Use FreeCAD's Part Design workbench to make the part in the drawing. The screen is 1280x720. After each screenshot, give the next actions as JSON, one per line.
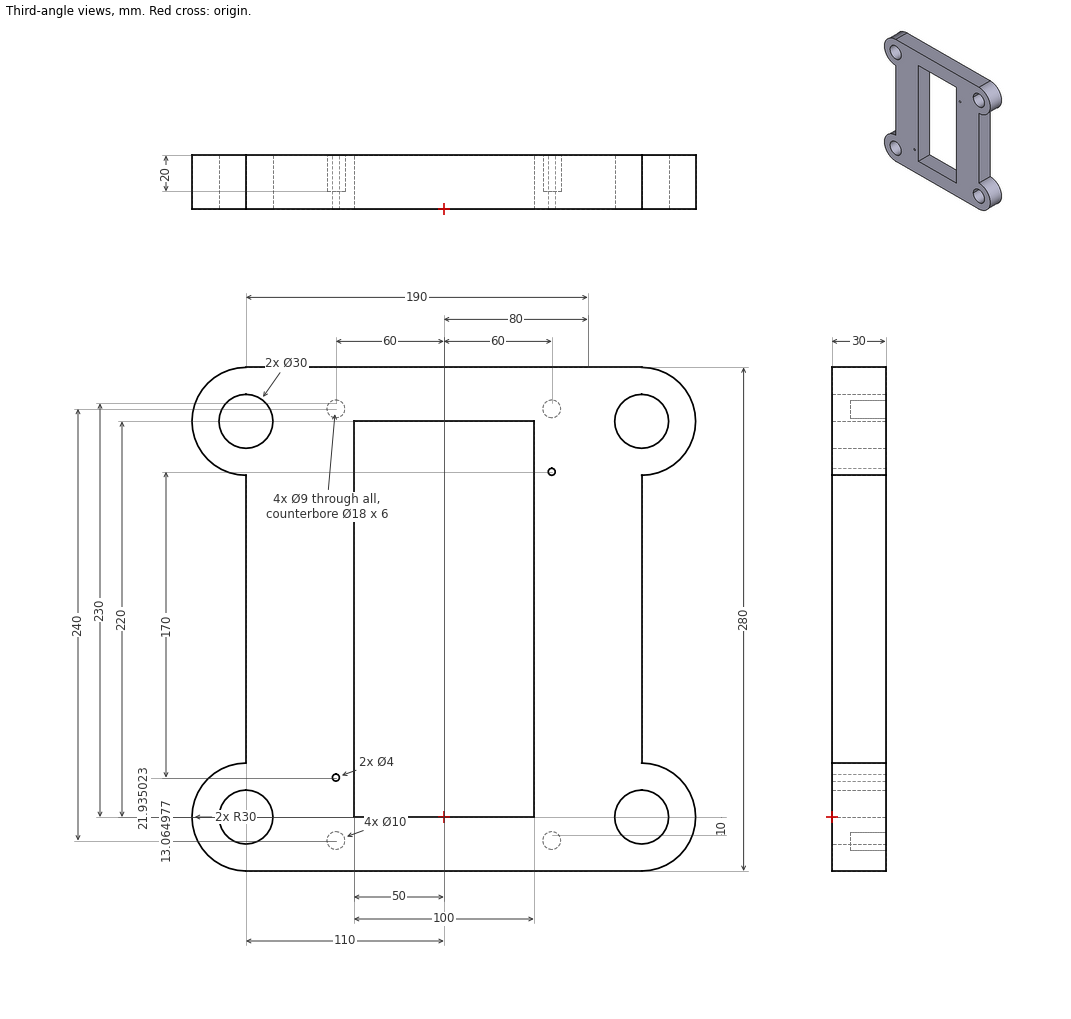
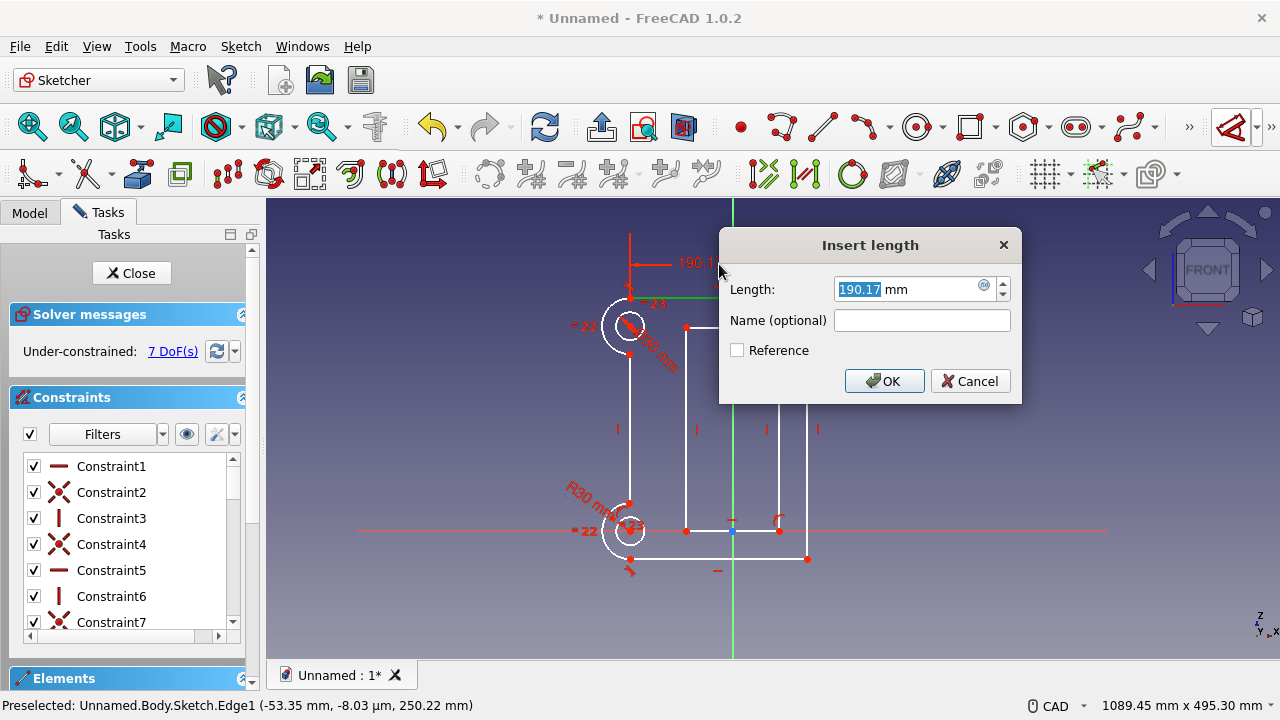
{"action": "type", "text": "190"}
{"action": "key", "text": "Return"}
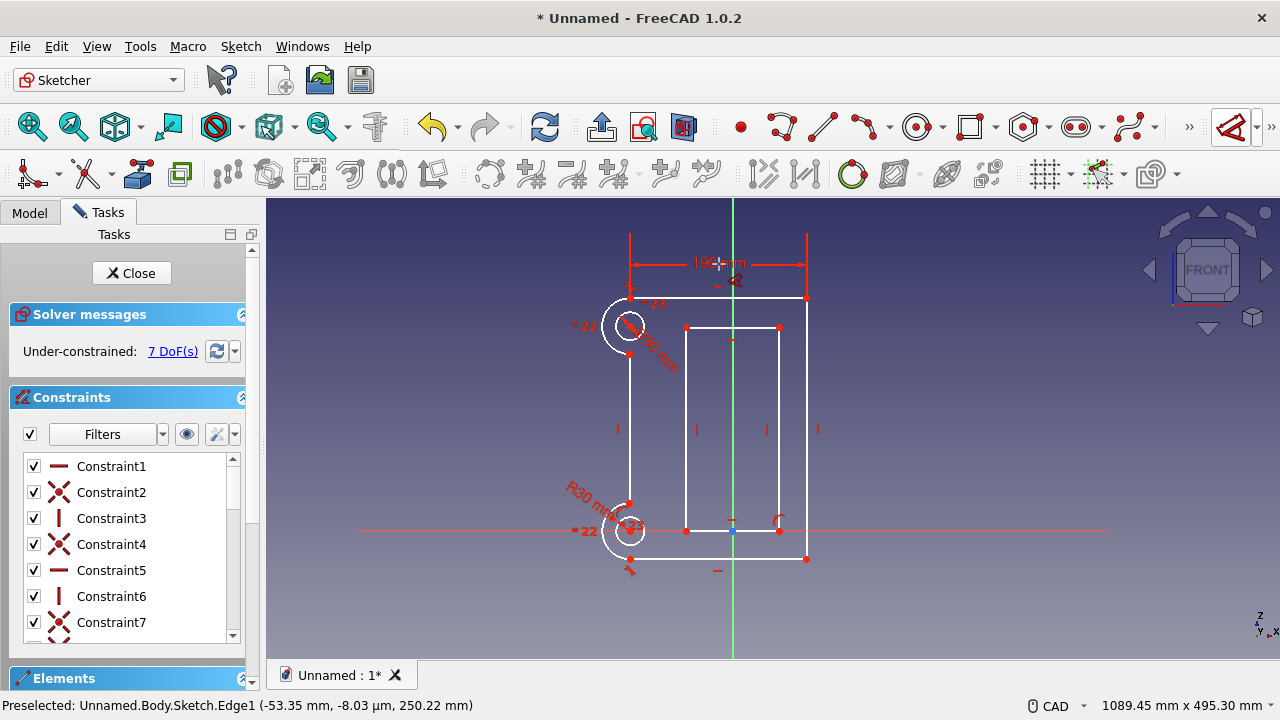
{"action": "left_click", "coordinate": [807, 377]}
{"action": "left_click", "coordinate": [841, 429]}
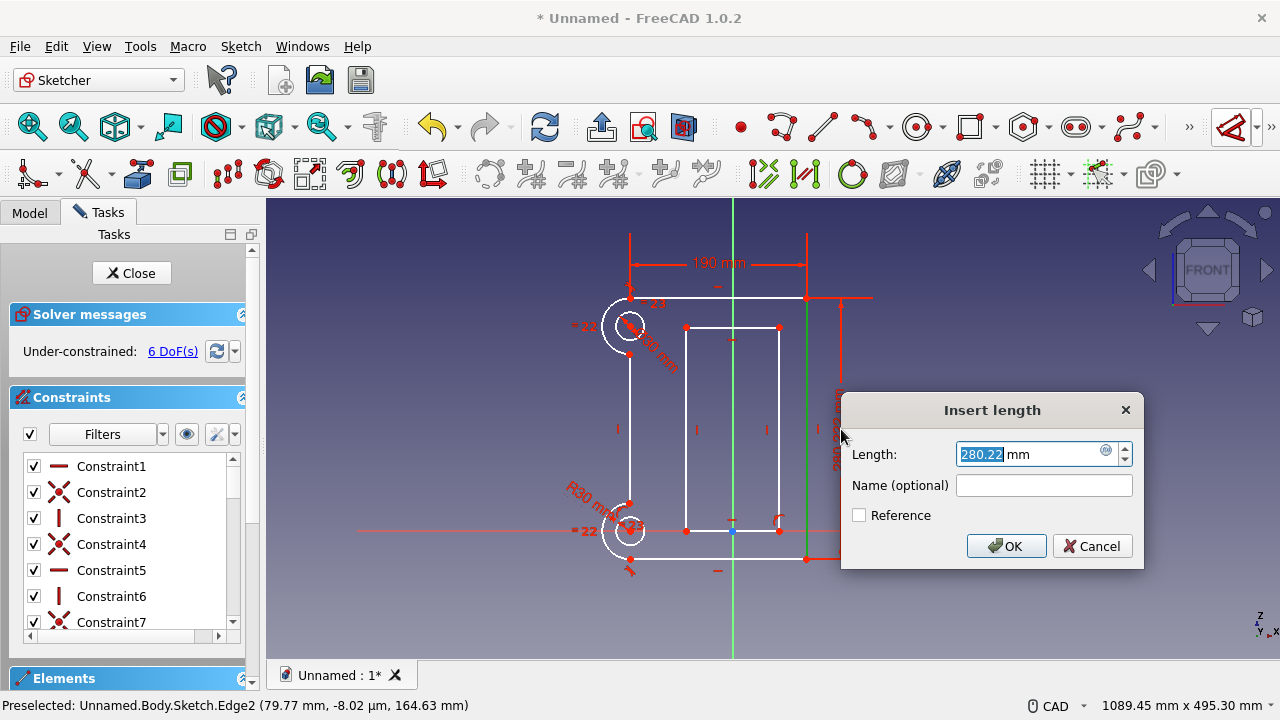
{"action": "type", "text": "280"}
{"action": "key", "text": "Return"}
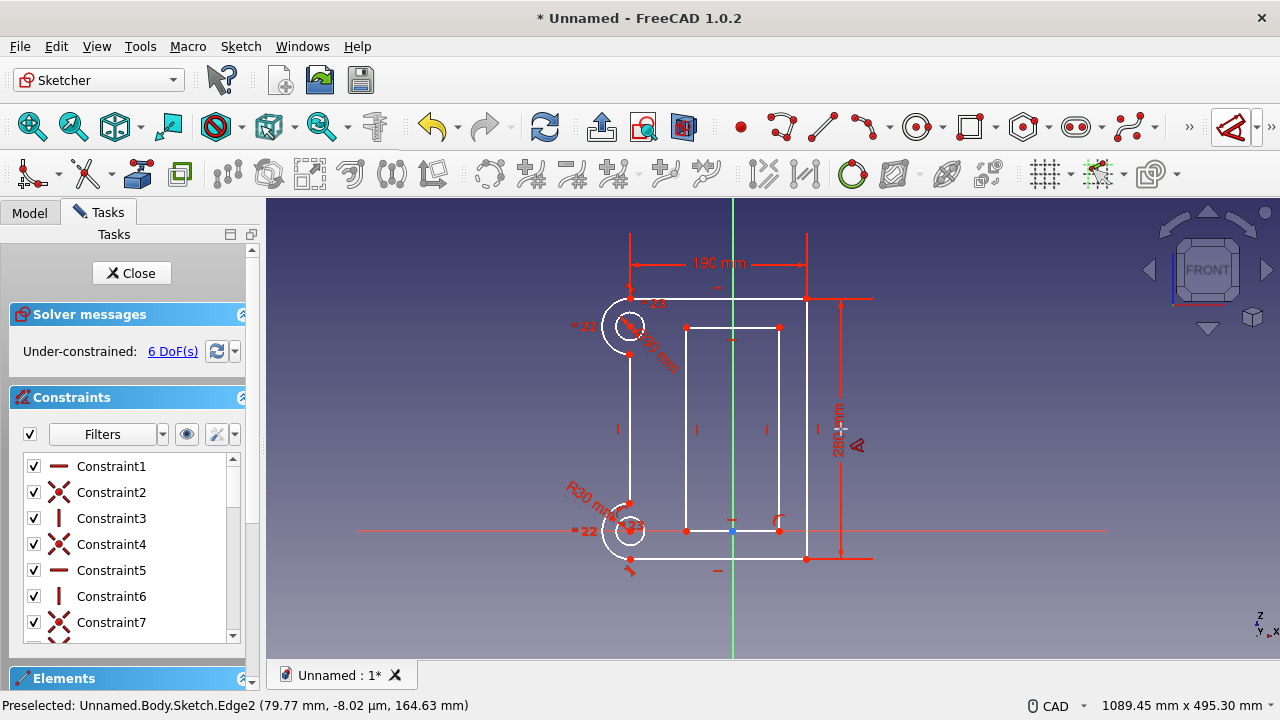
{"action": "left_click", "coordinate": [754, 559]}
{"action": "left_click", "coordinate": [719, 593]}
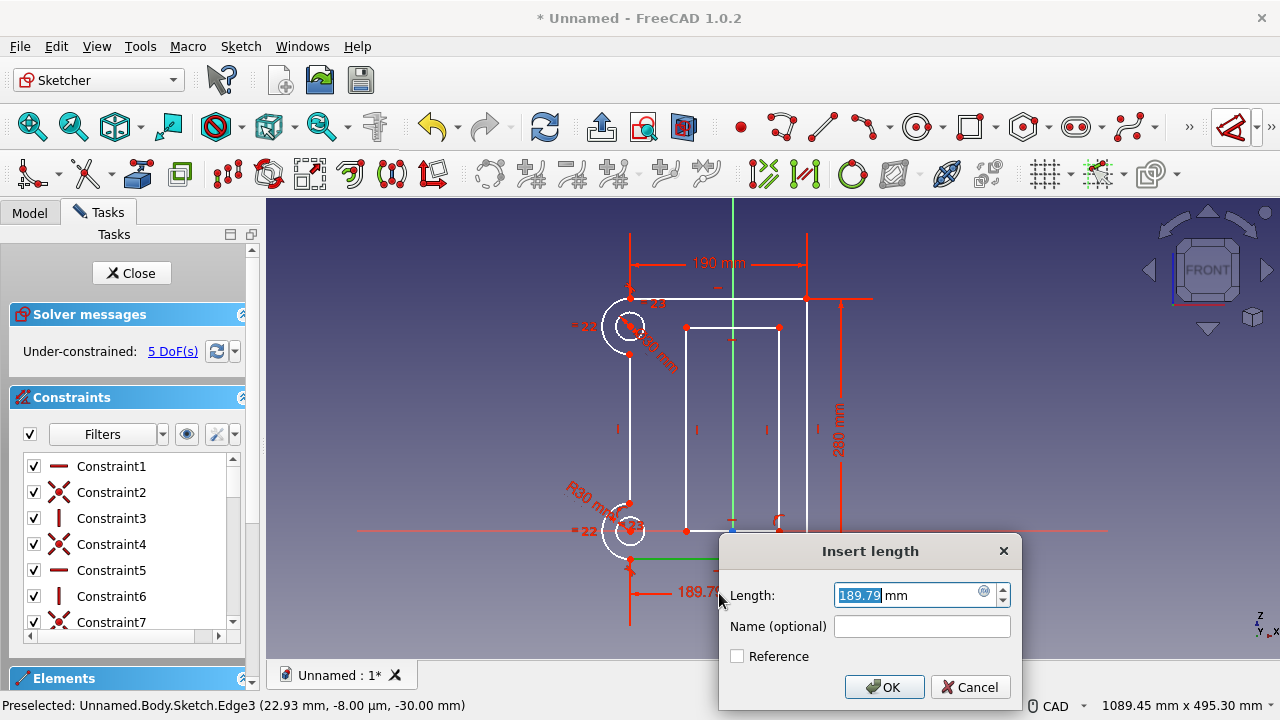
{"action": "type", "text": "190"}
{"action": "key", "text": "Return"}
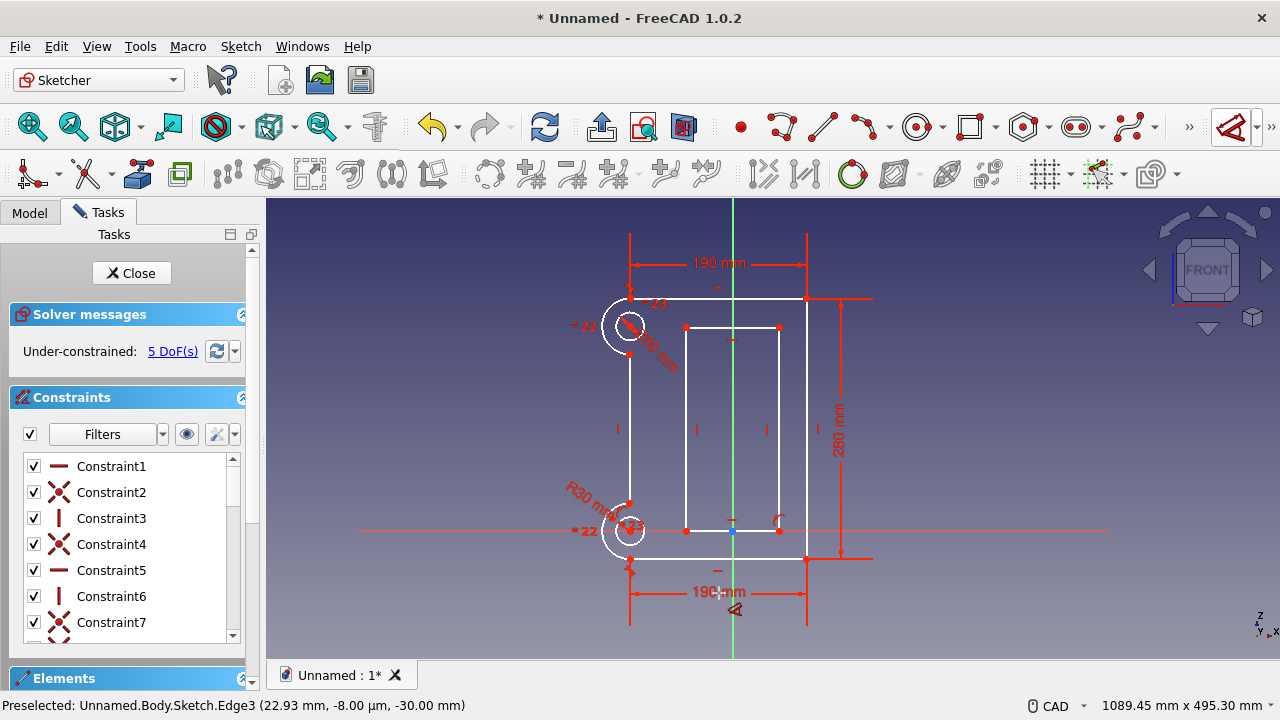
{"action": "left_click", "coordinate": [686, 389]}
{"action": "left_click", "coordinate": [652, 429]}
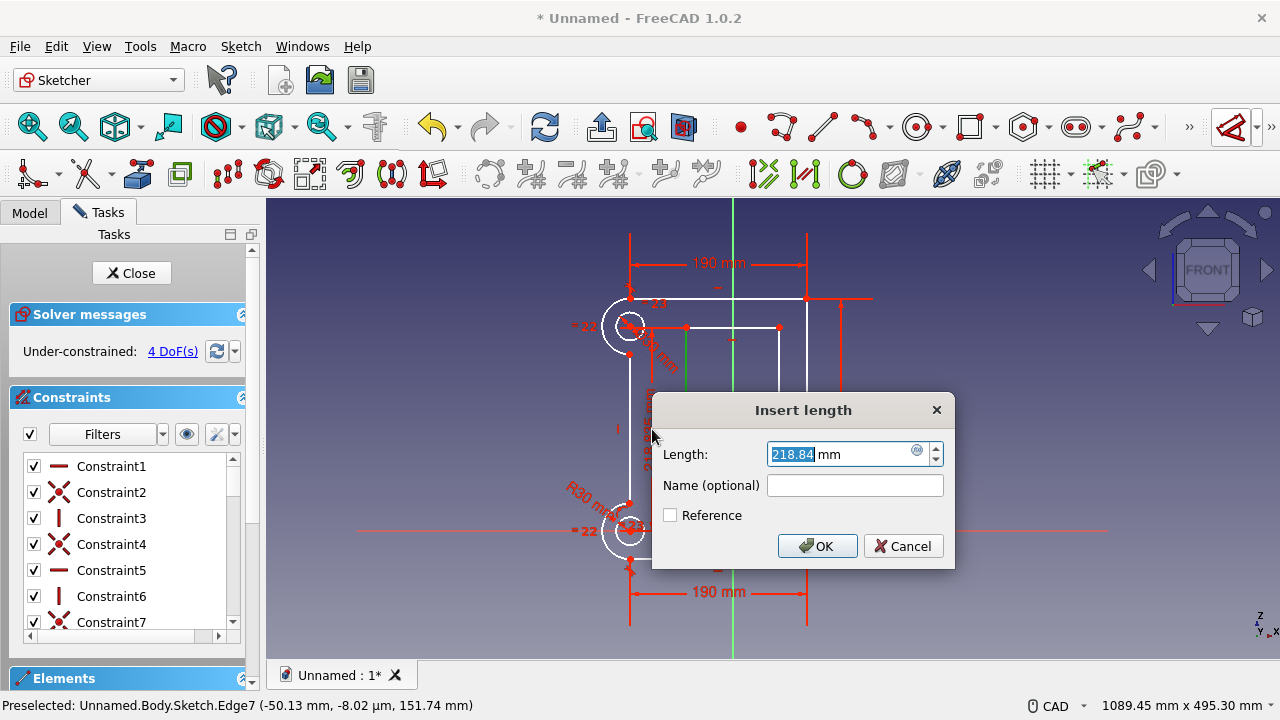
{"action": "type", "text": "220"}
{"action": "key", "text": "Return"}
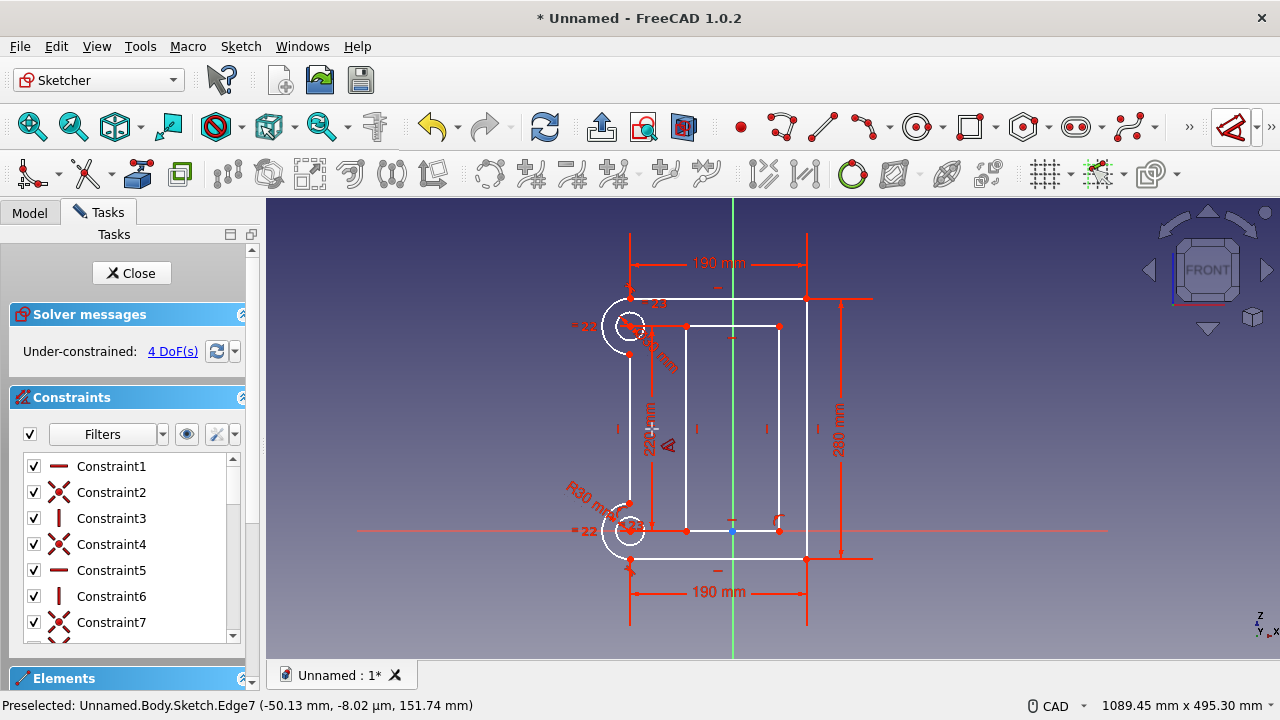
{"action": "left_click", "coordinate": [714, 531]}
{"action": "left_click", "coordinate": [711, 497]}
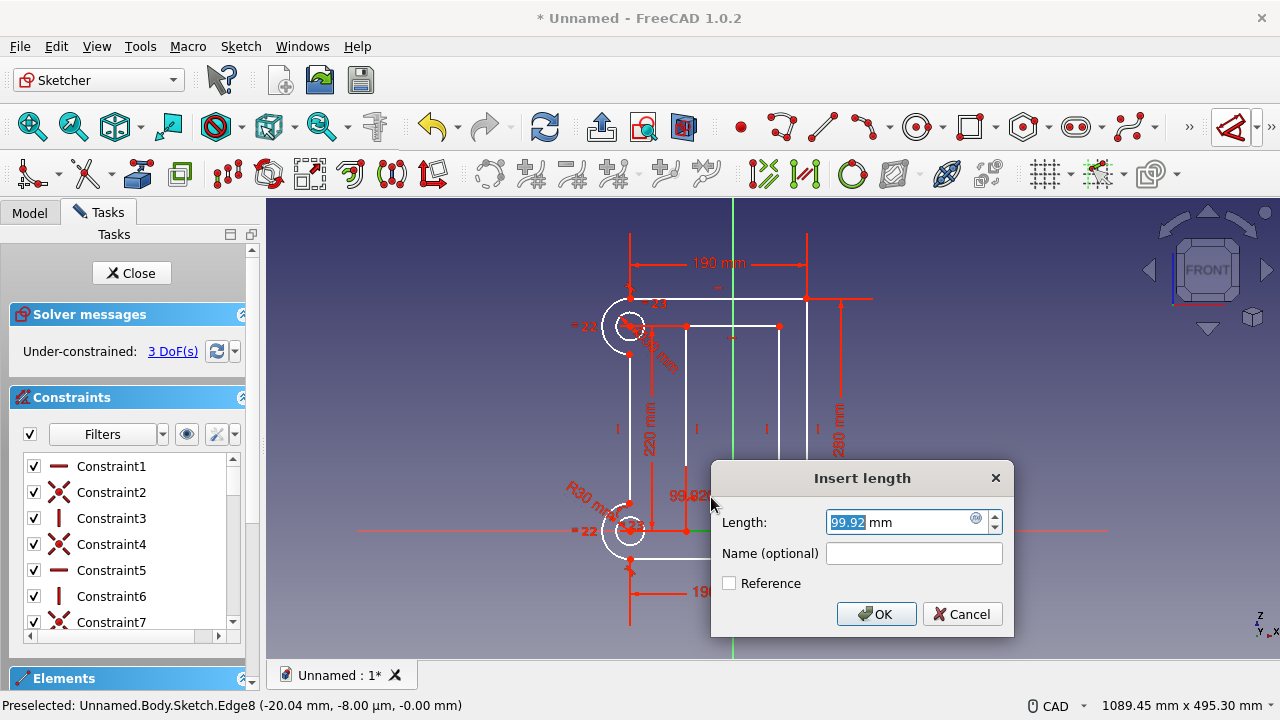
{"action": "type", "text": "100"}
{"action": "key", "text": "Return"}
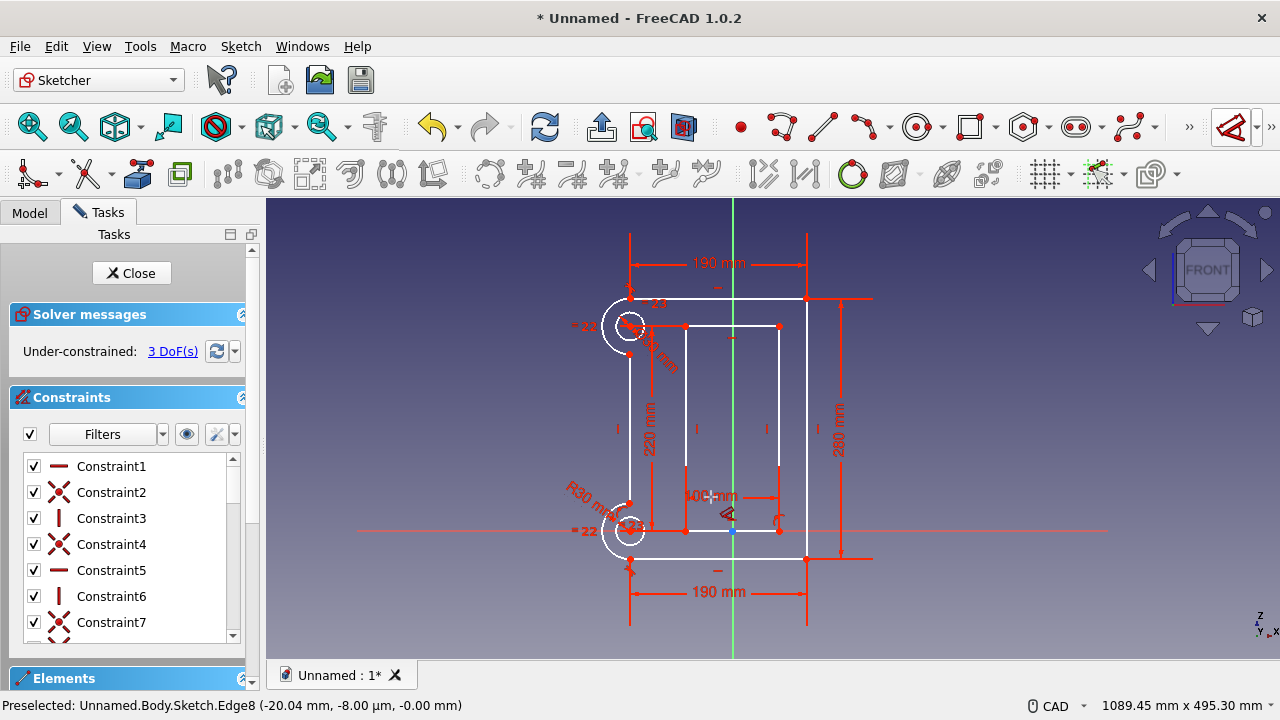
{"action": "left_click", "coordinate": [807, 299]}
{"action": "left_click", "coordinate": [796, 265]}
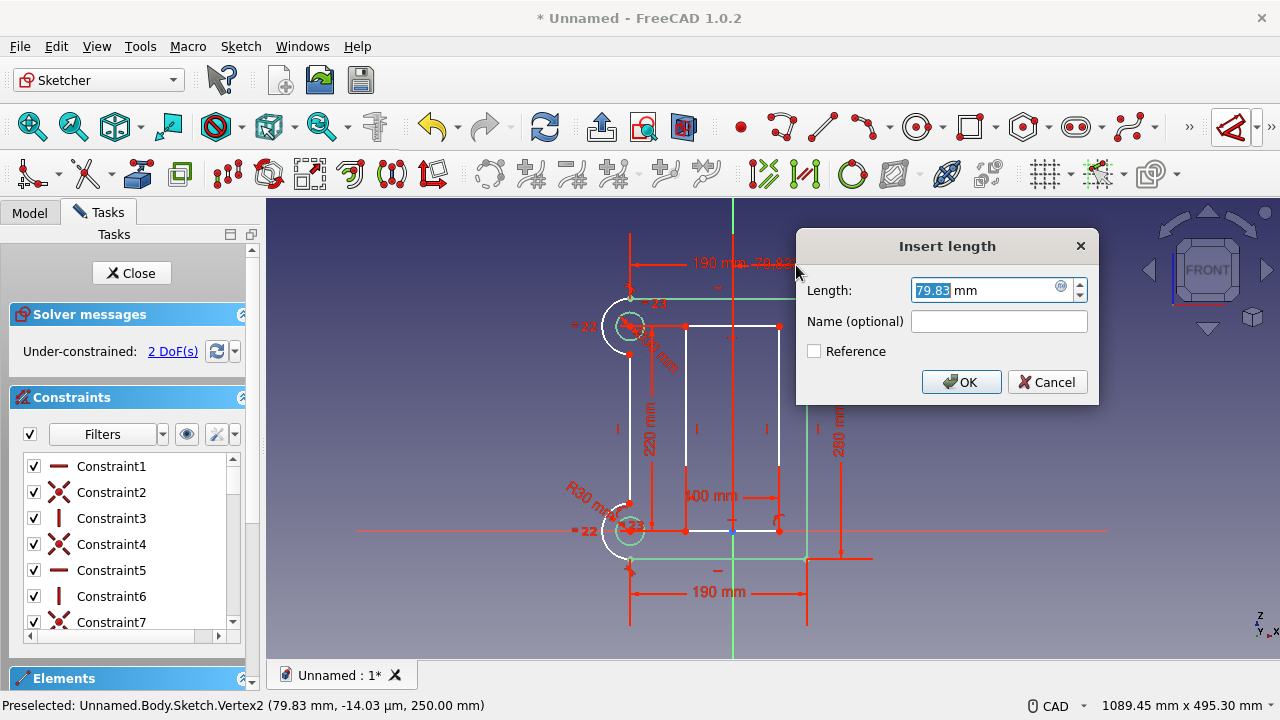
{"action": "type", "text": "80"}
{"action": "key", "text": "Return"}